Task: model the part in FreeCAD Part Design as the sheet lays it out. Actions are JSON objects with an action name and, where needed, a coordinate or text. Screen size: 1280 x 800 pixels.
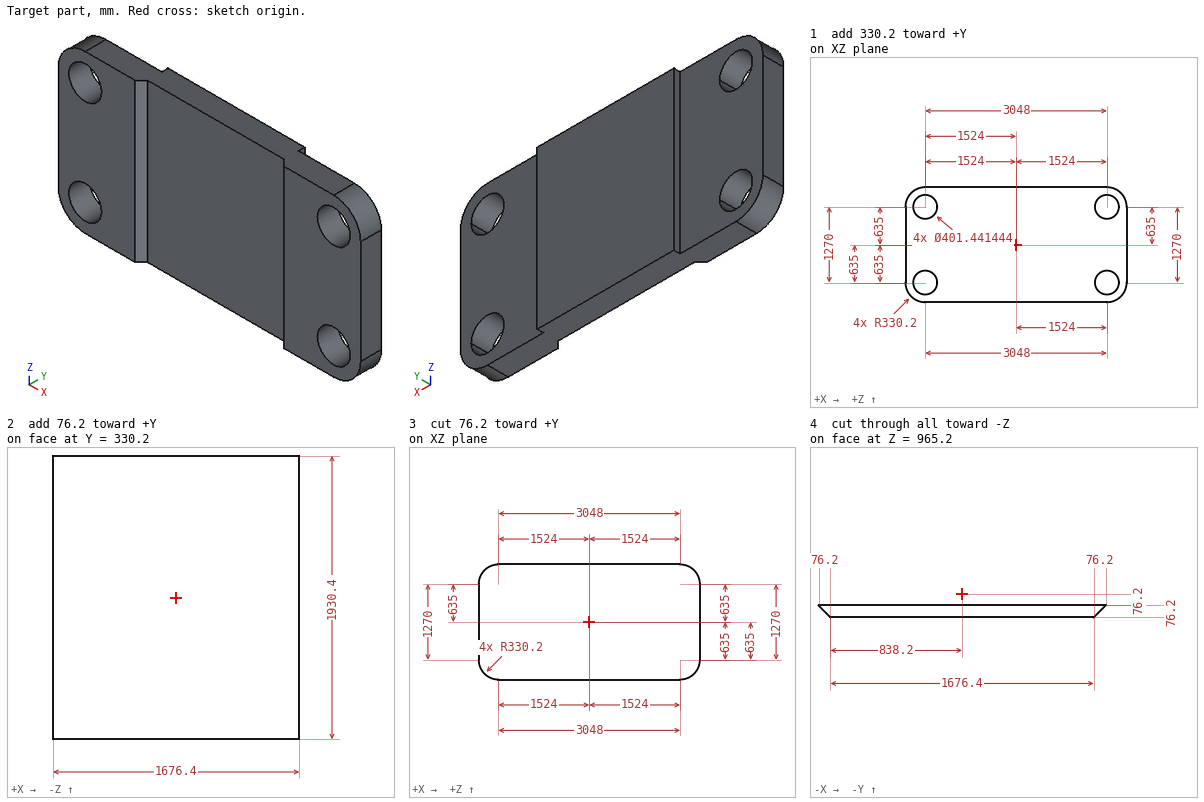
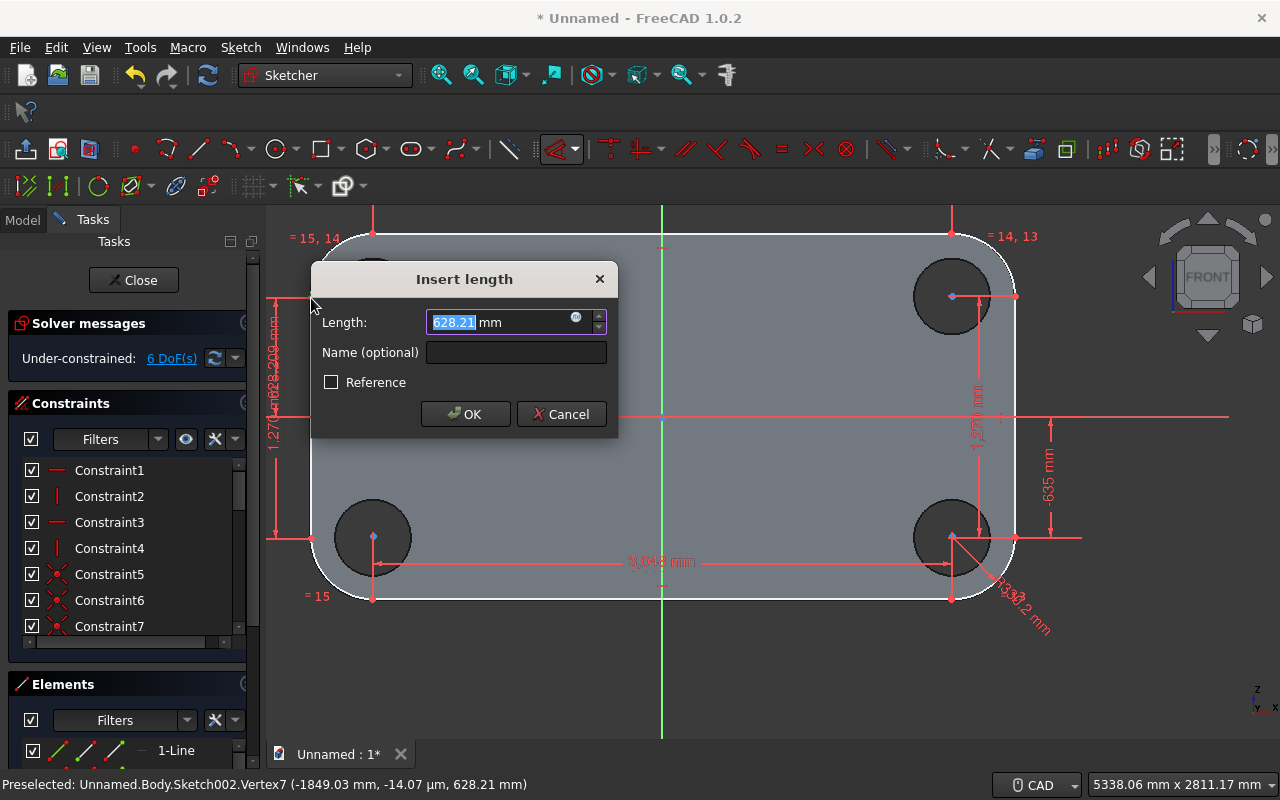
{"action": "type", "text": "635"}
{"action": "key", "text": "Return"}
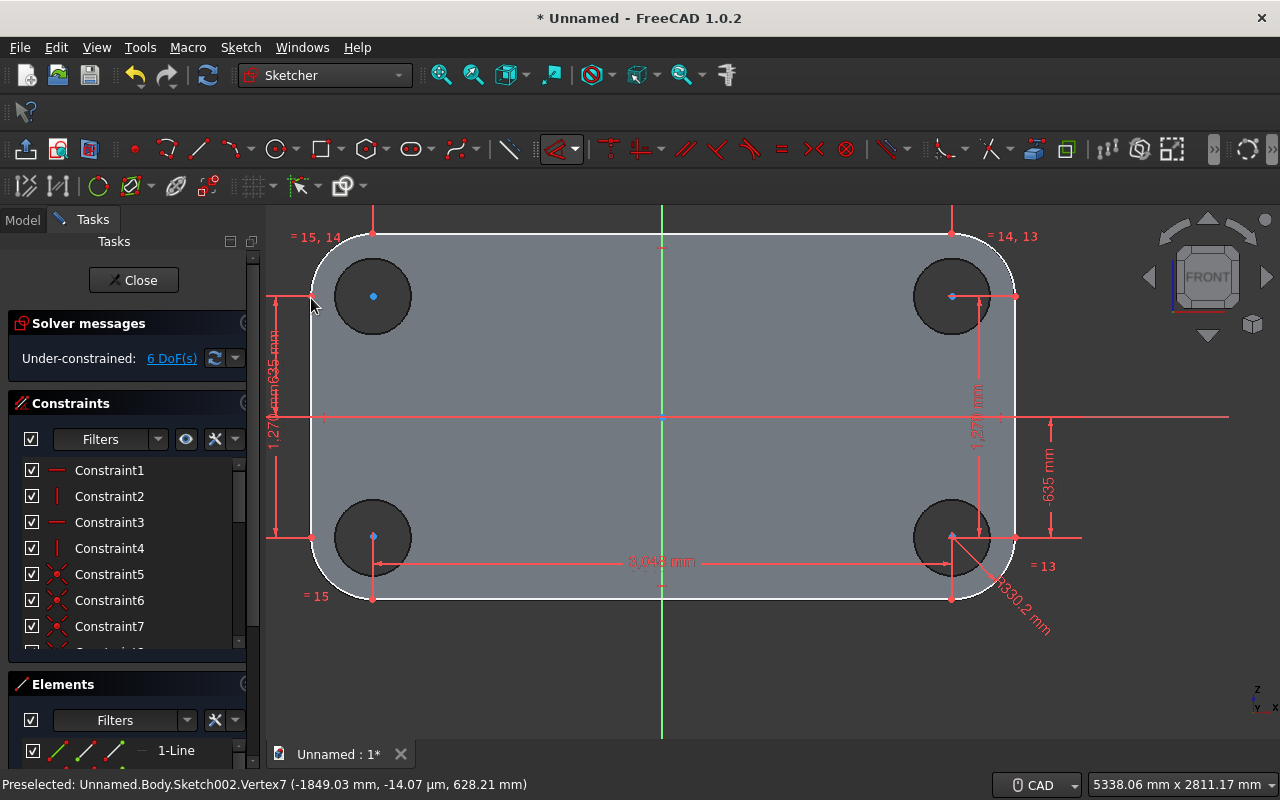
{"action": "left_click", "coordinate": [952, 537]}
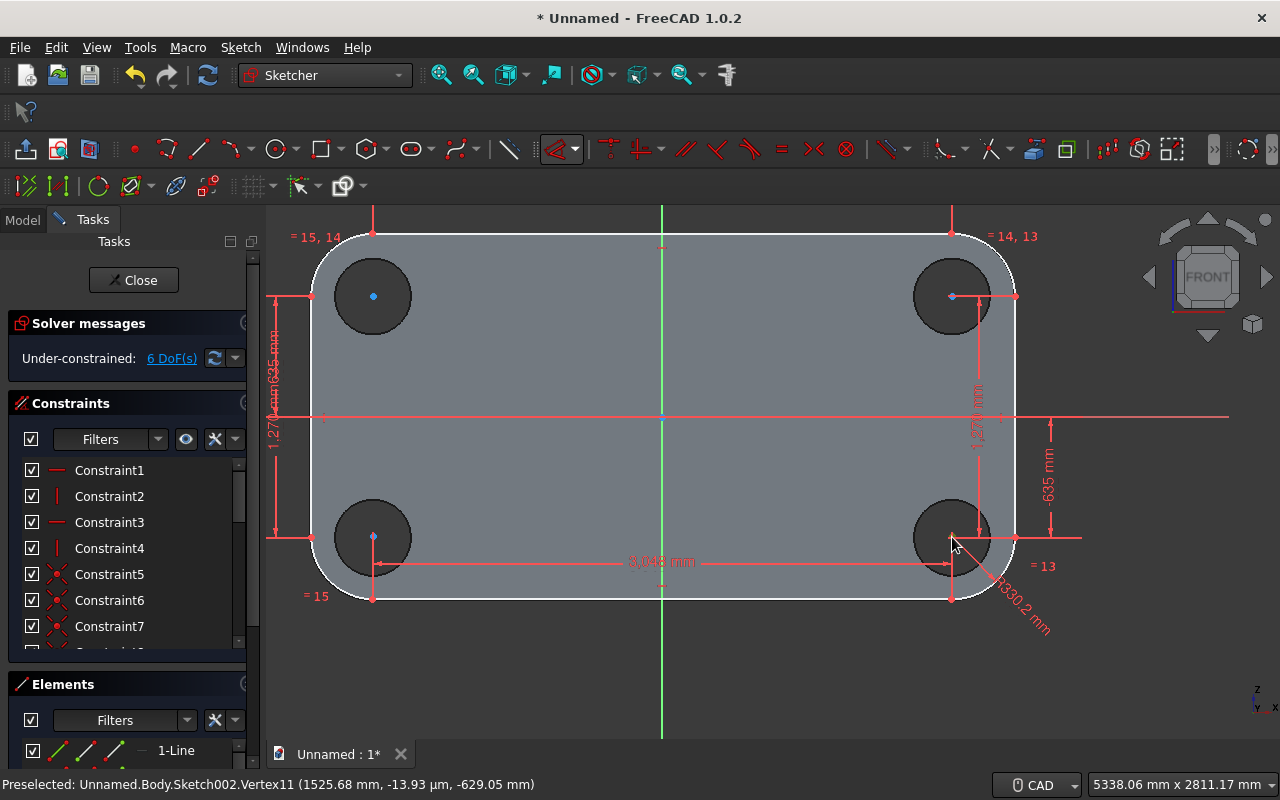
{"action": "key", "text": "i"}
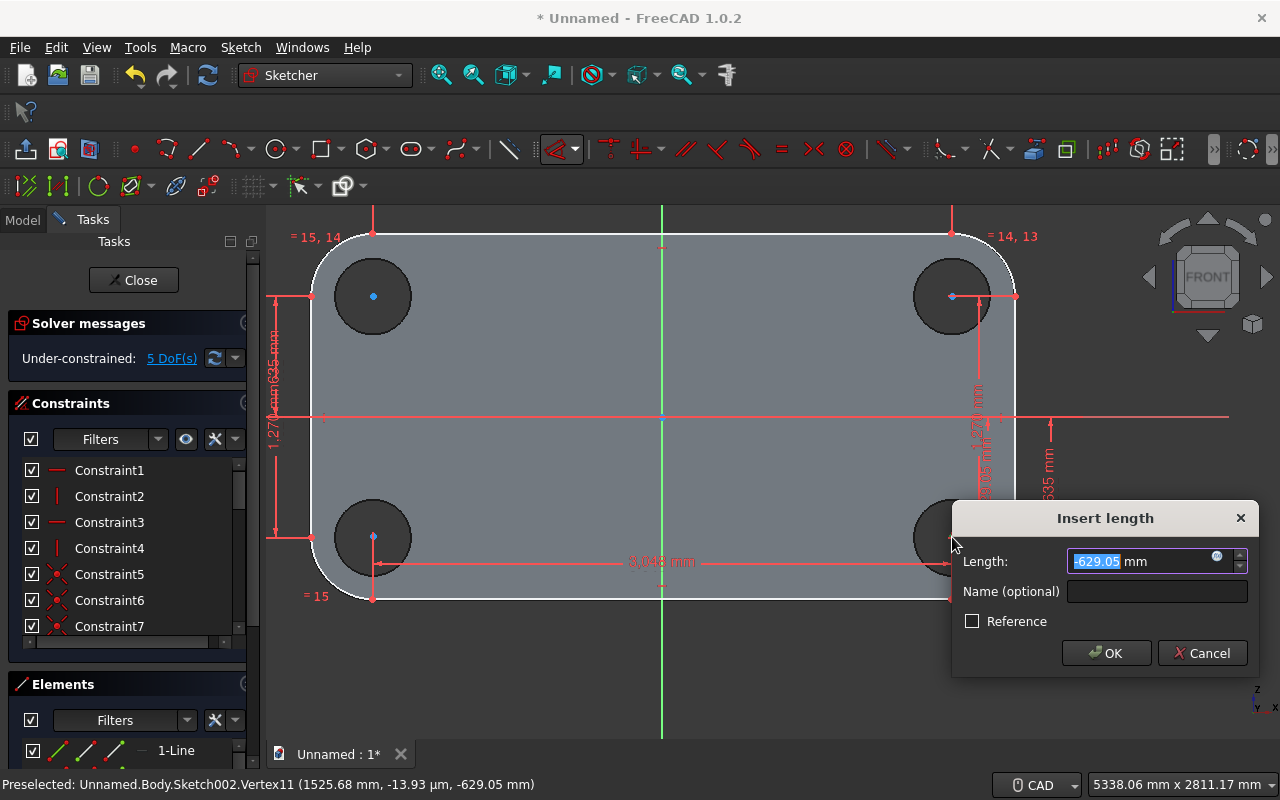
{"action": "type", "text": "-635"}
{"action": "key", "text": "Return"}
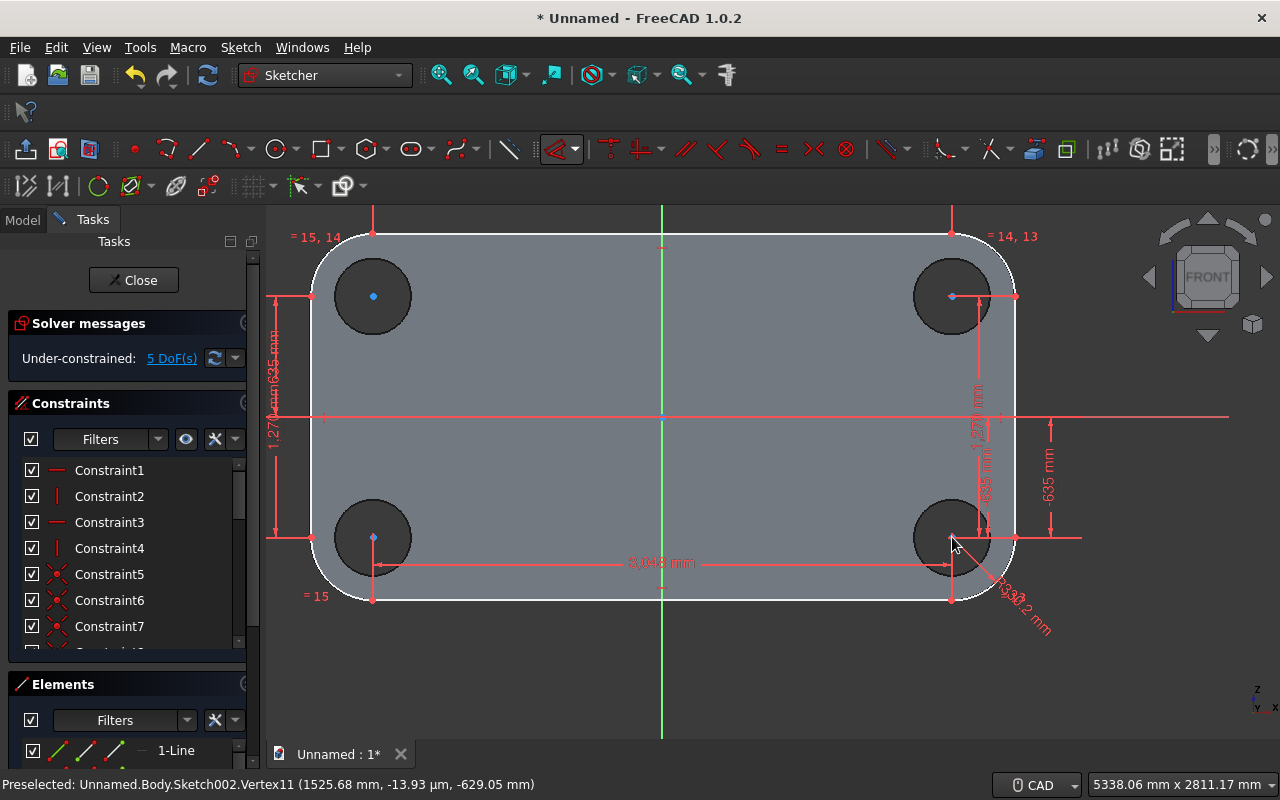
{"action": "left_click", "coordinate": [952, 297]}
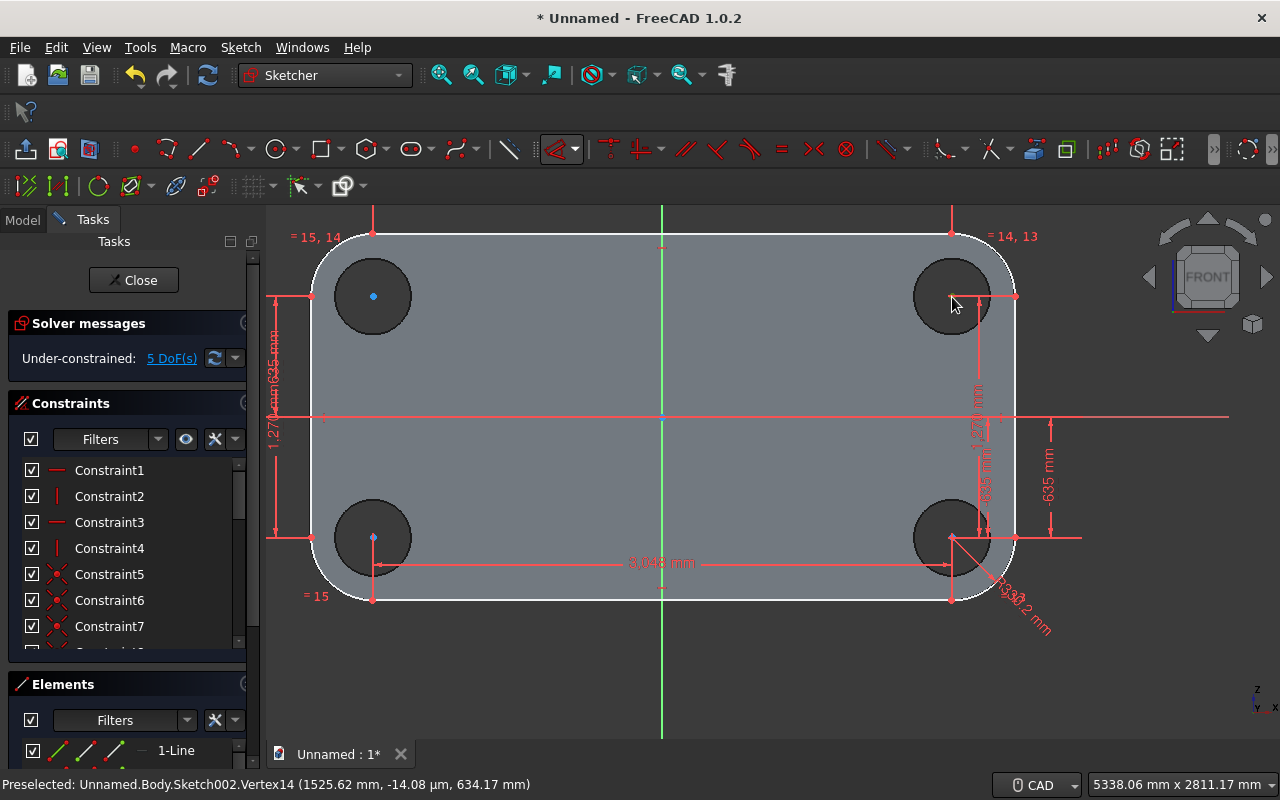
{"action": "key", "text": "i"}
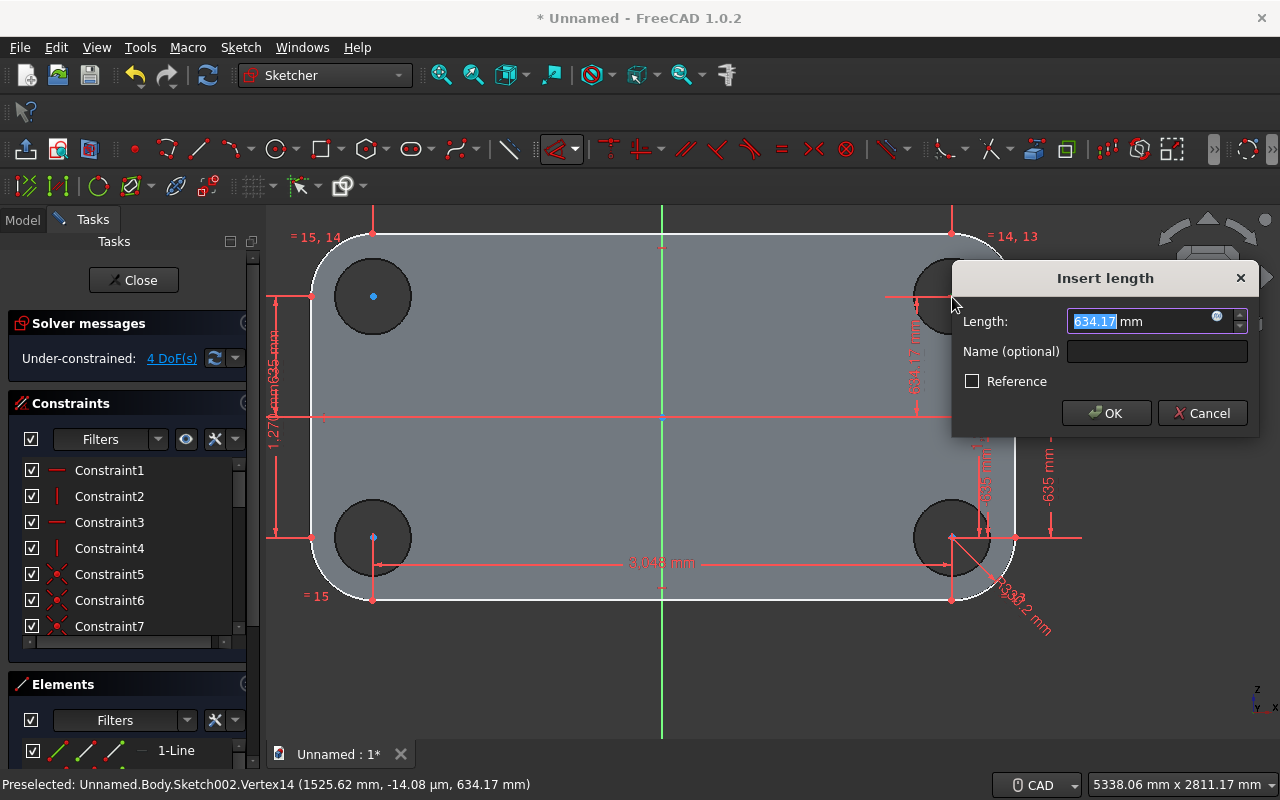
{"action": "type", "text": "635"}
{"action": "key", "text": "Return"}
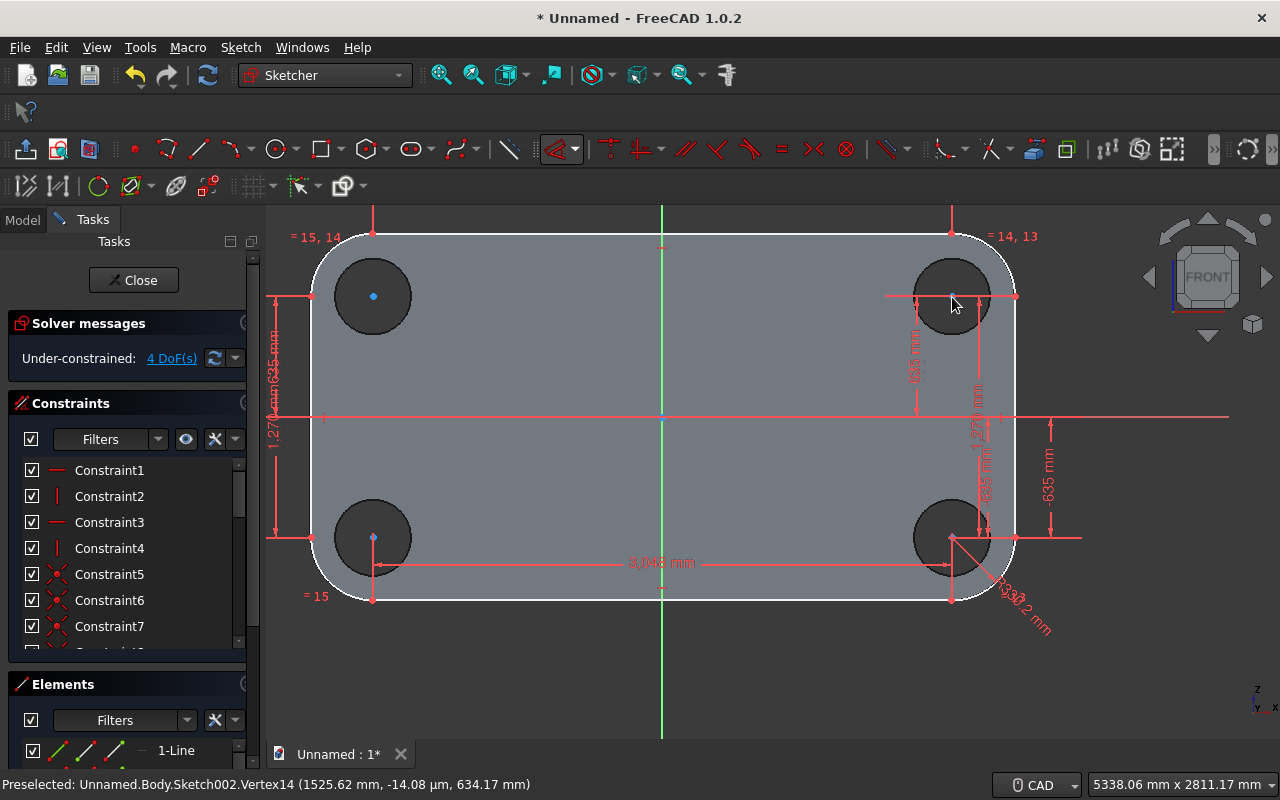
{"action": "left_click", "coordinate": [373, 600]}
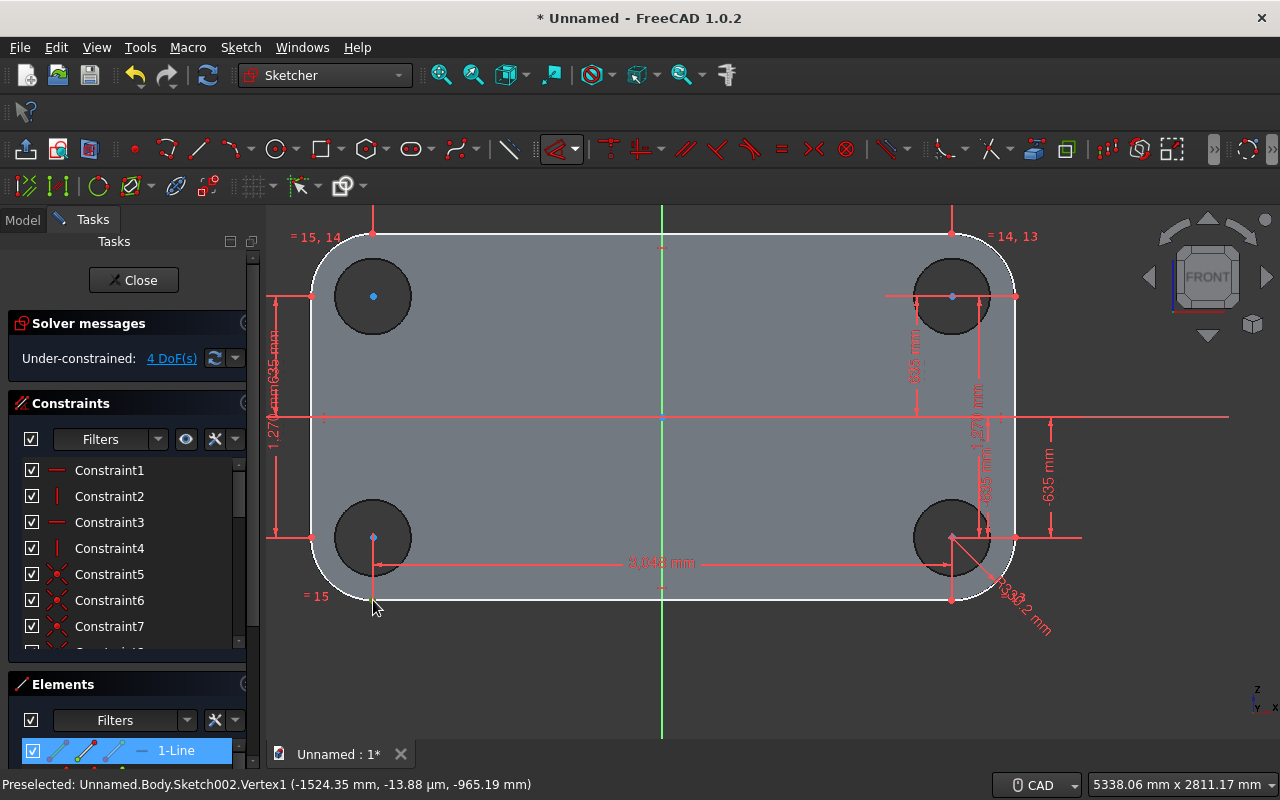
{"action": "key", "text": "l"}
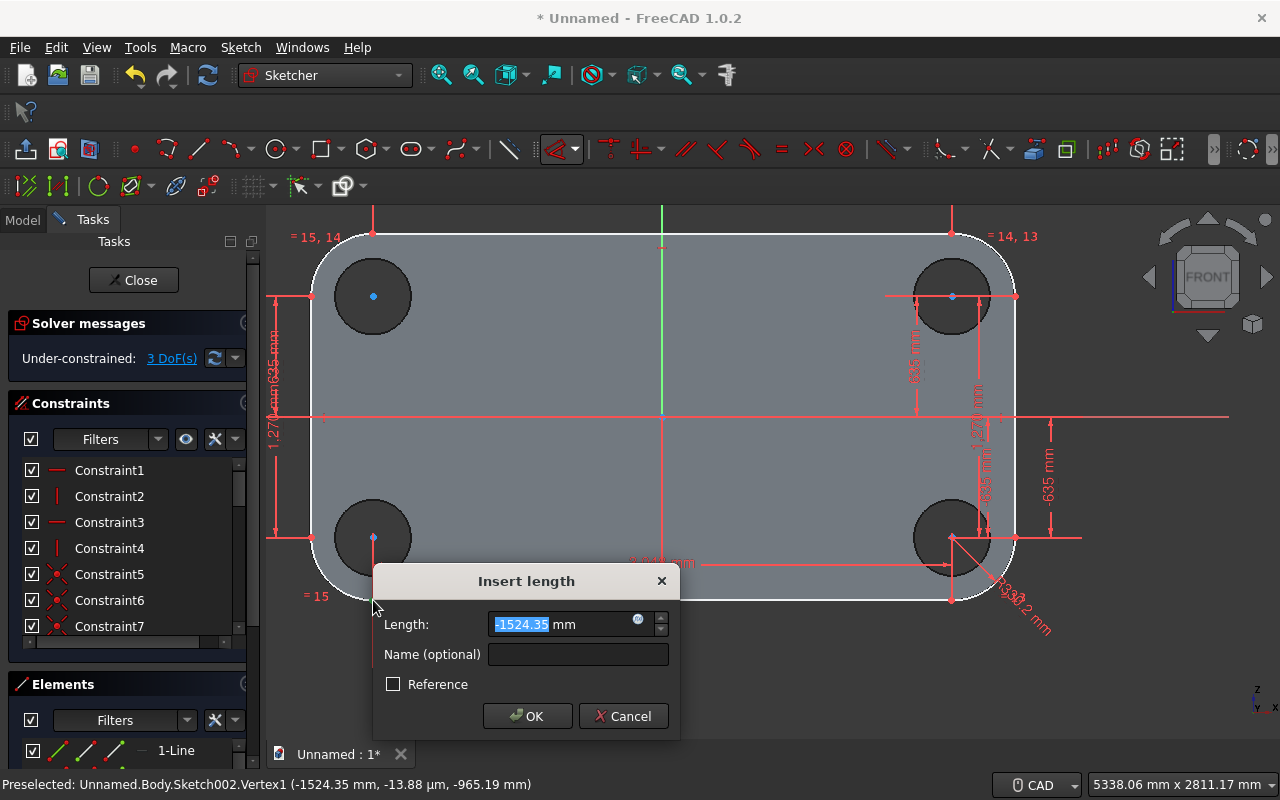
{"action": "type", "text": "-1524"}
{"action": "key", "text": "Return"}